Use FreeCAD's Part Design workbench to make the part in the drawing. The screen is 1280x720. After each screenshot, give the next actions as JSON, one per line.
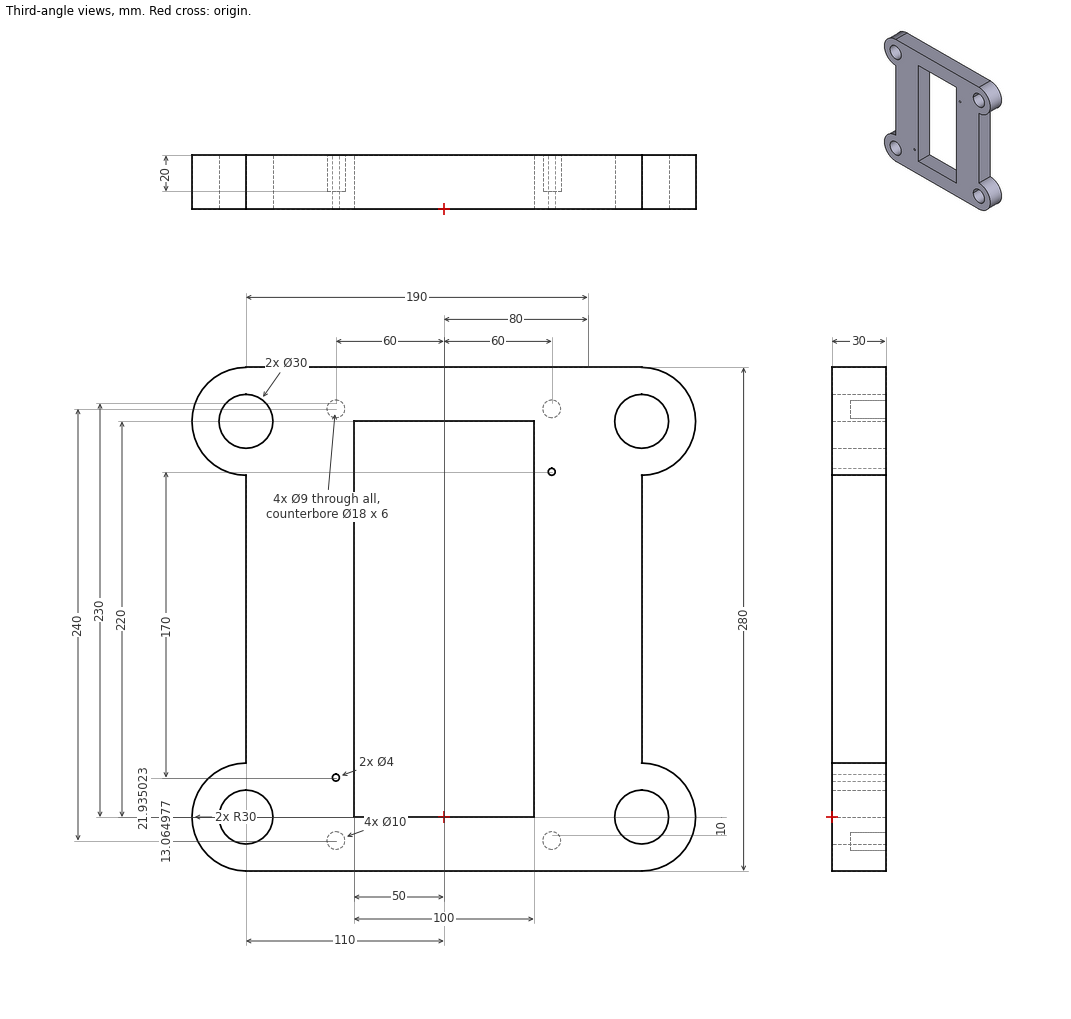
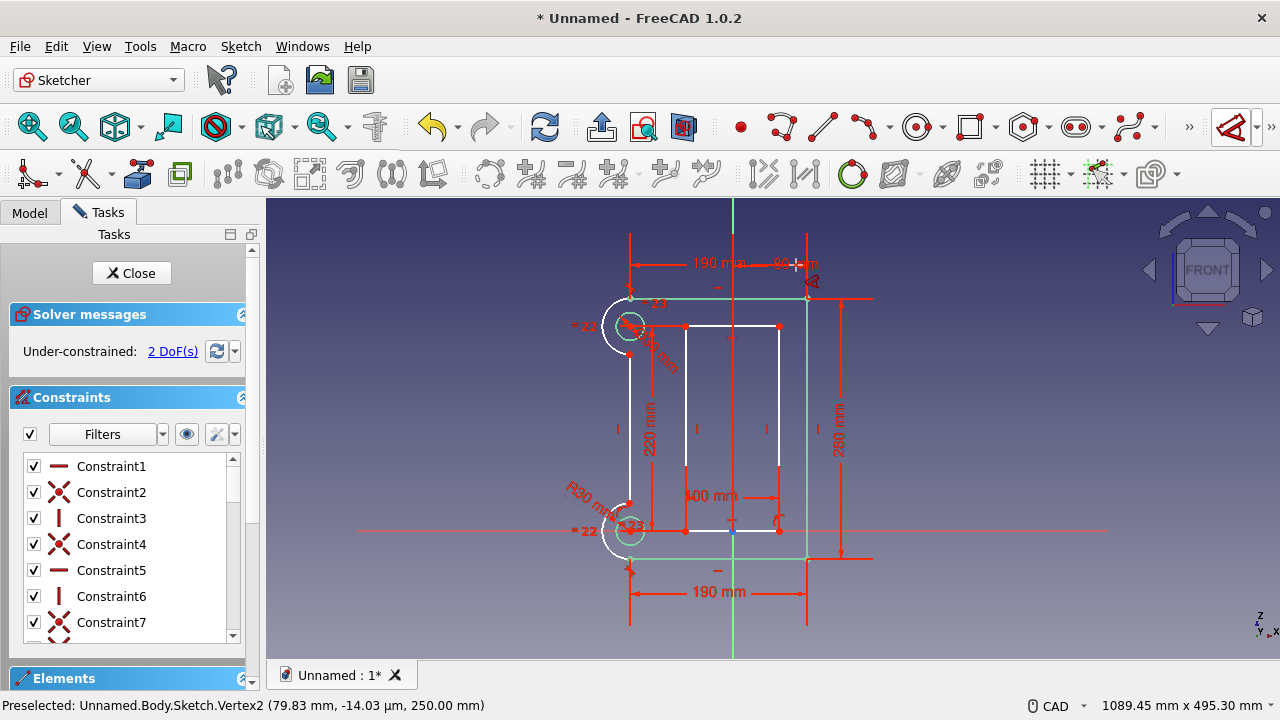
{"action": "left_click", "coordinate": [686, 326]}
{"action": "left_click", "coordinate": [709, 613]}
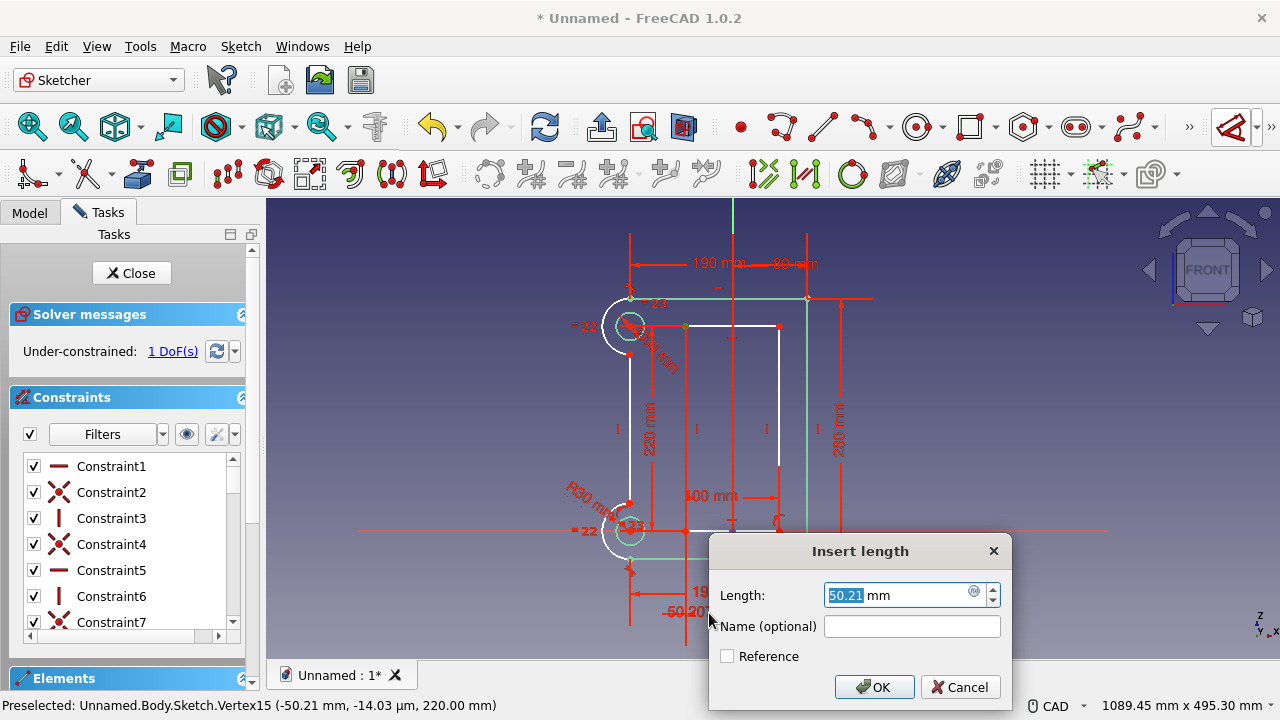
{"action": "type", "text": "50"}
{"action": "key", "text": "Return"}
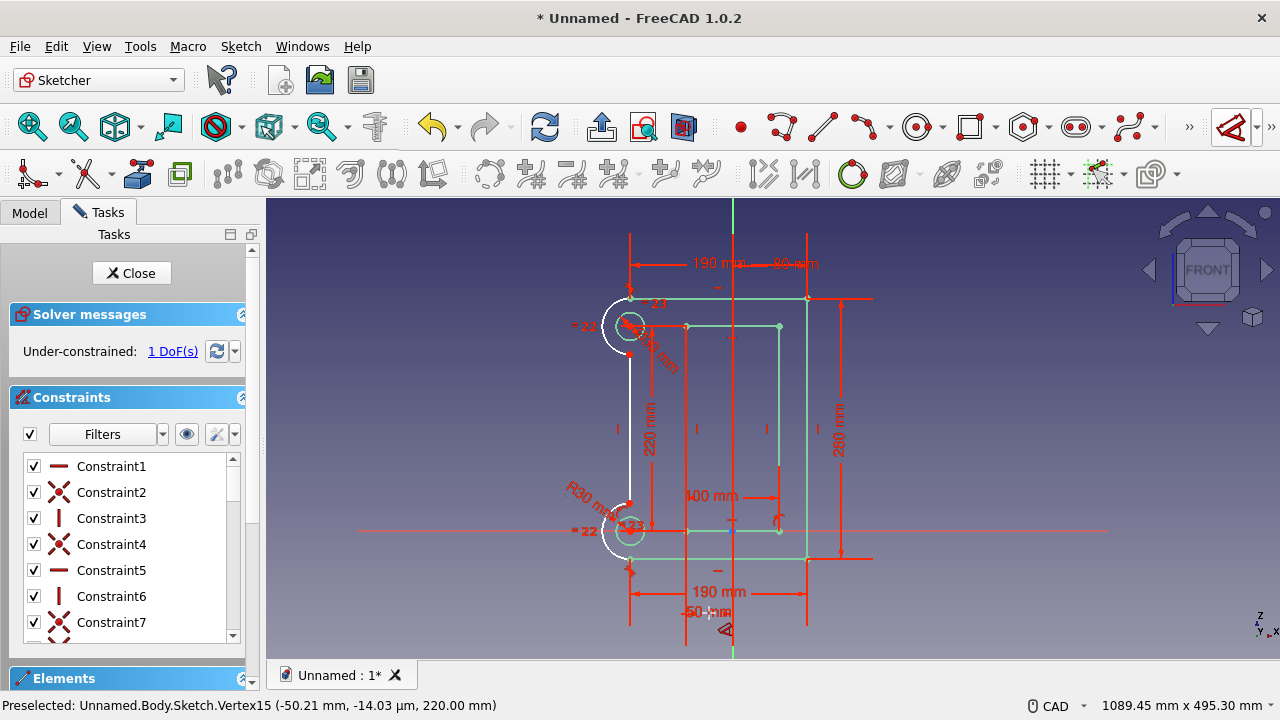
{"action": "left_click", "coordinate": [630, 503]}
{"action": "left_click", "coordinate": [658, 469]}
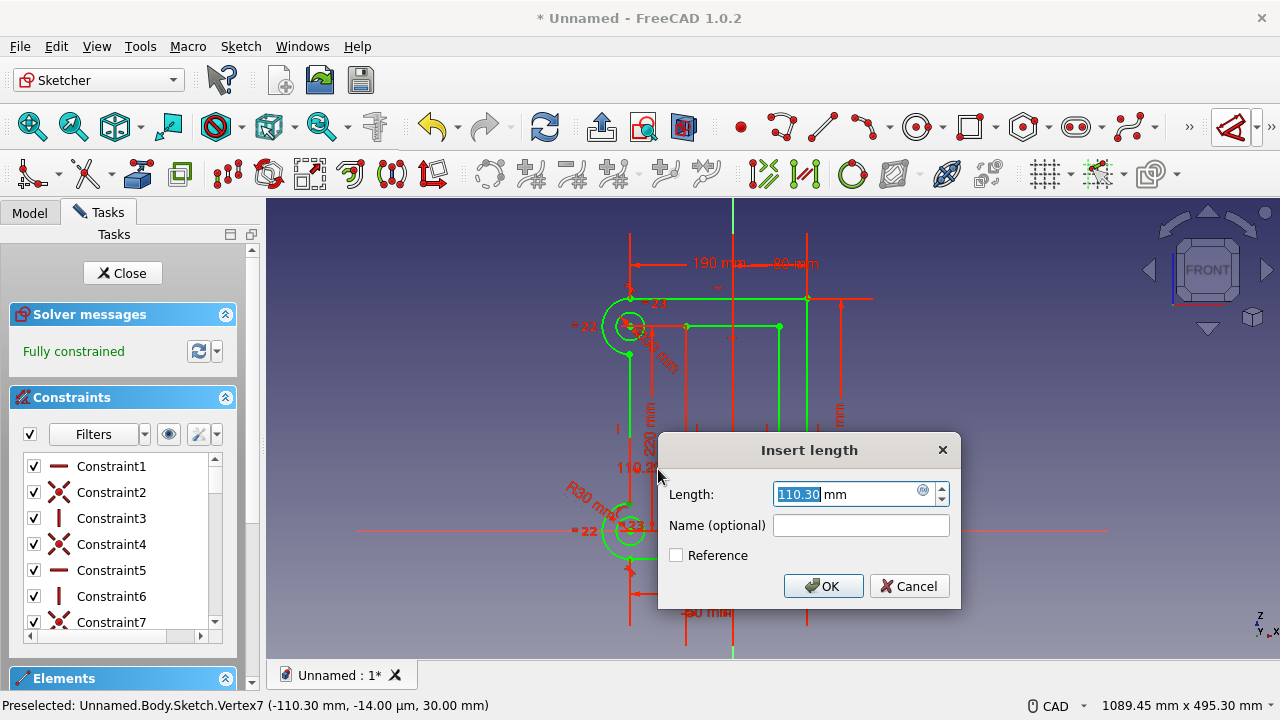
{"action": "type", "text": "110"}
{"action": "key", "text": "Return"}
{"action": "key", "text": "Escape"}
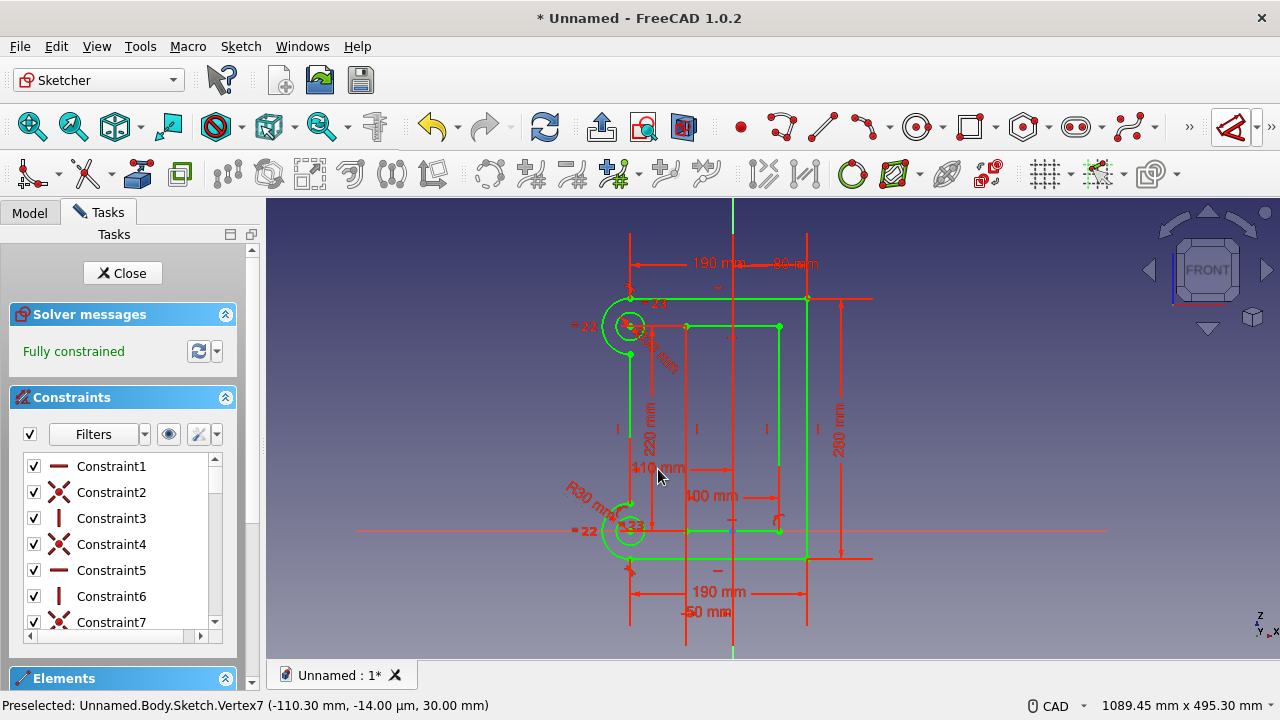
{"action": "left_click", "coordinate": [123, 273]}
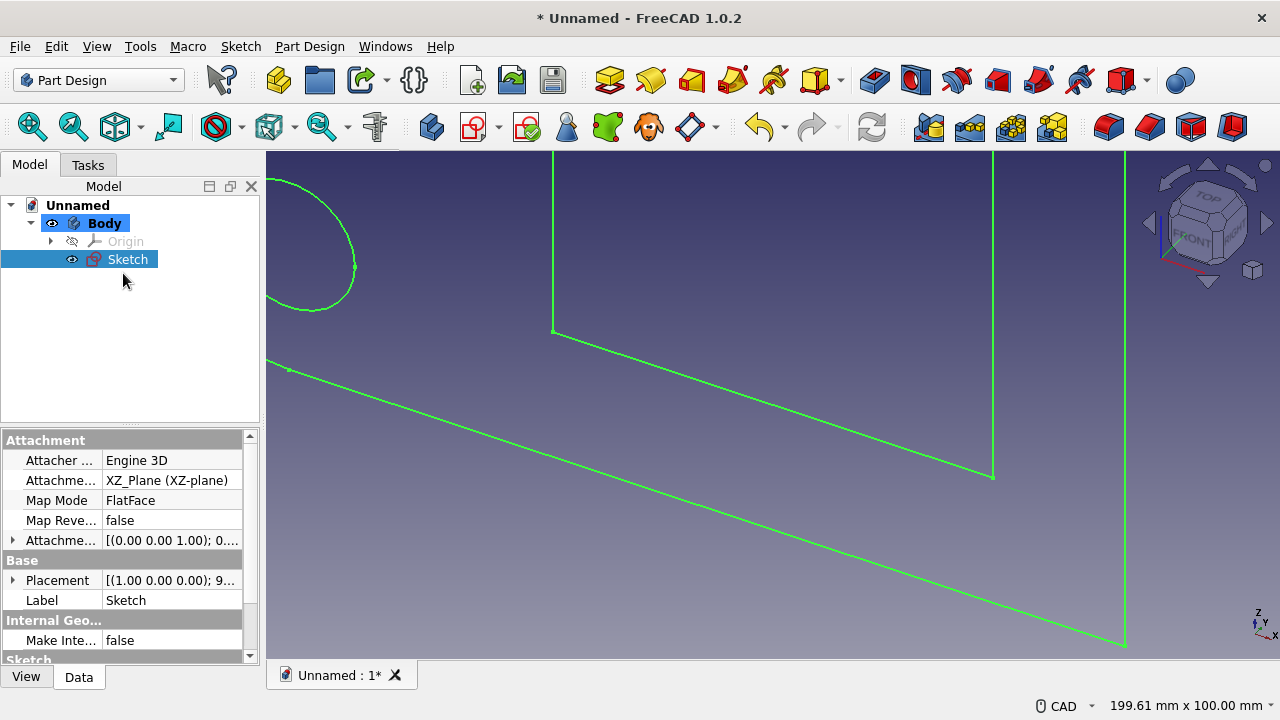
{"action": "left_click", "coordinate": [610, 80]}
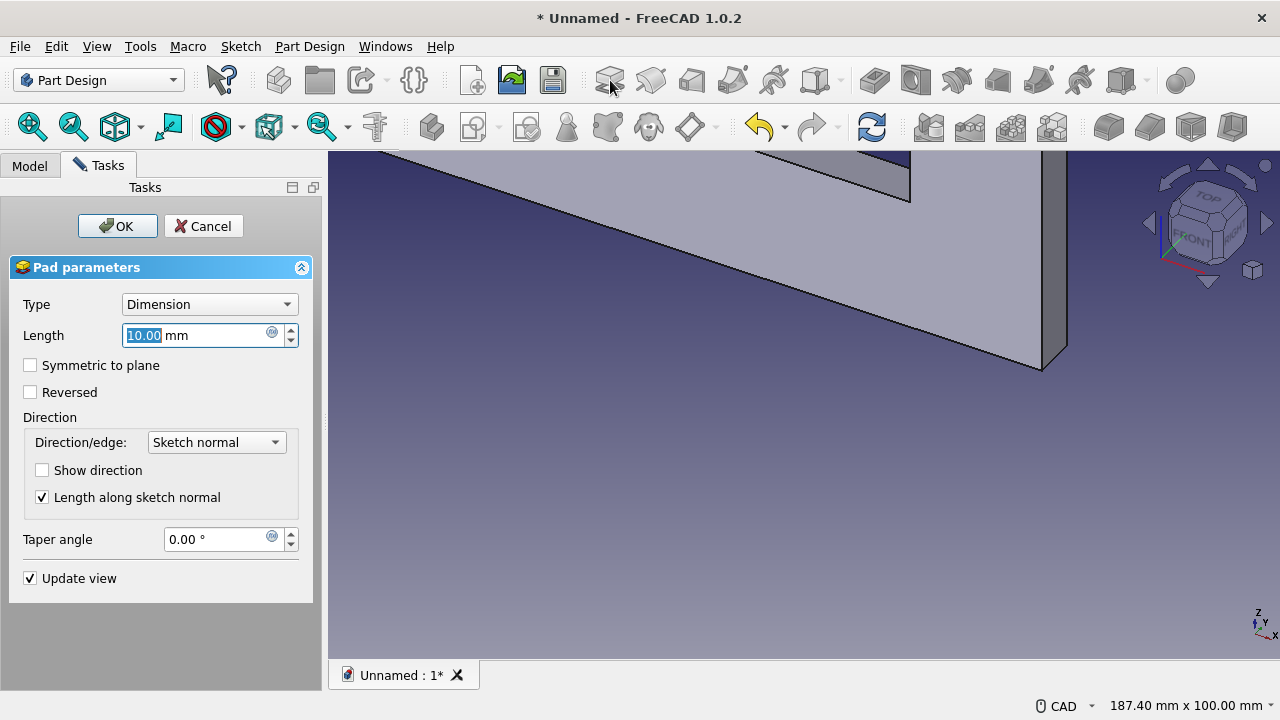
{"action": "type", "text": "30"}
{"action": "key", "text": "Tab"}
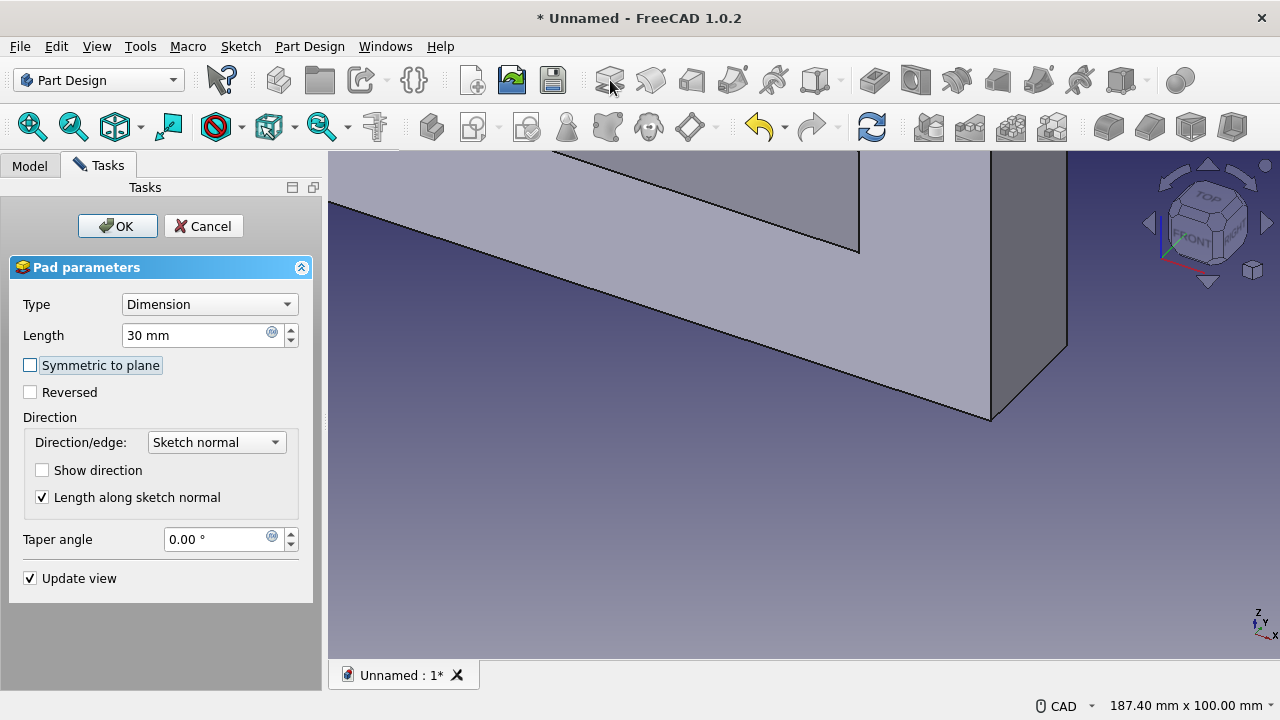
{"action": "left_click", "coordinate": [31, 392]}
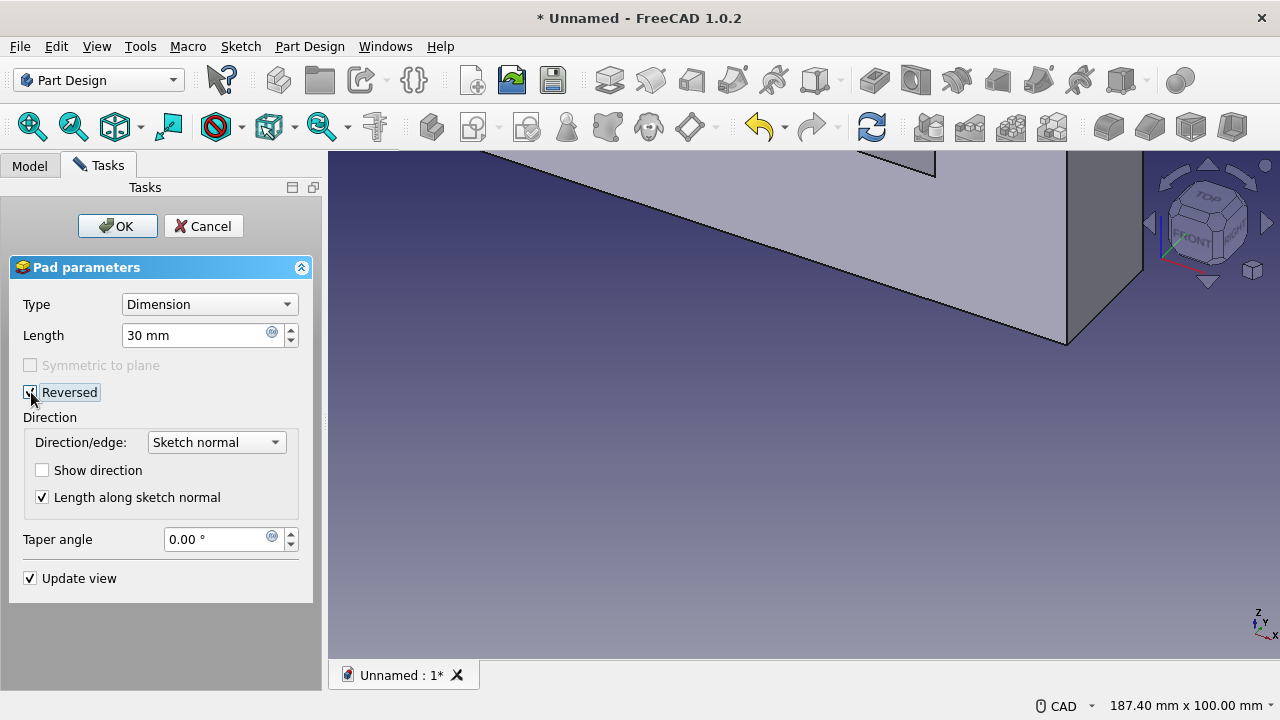
{"action": "left_click", "coordinate": [118, 226]}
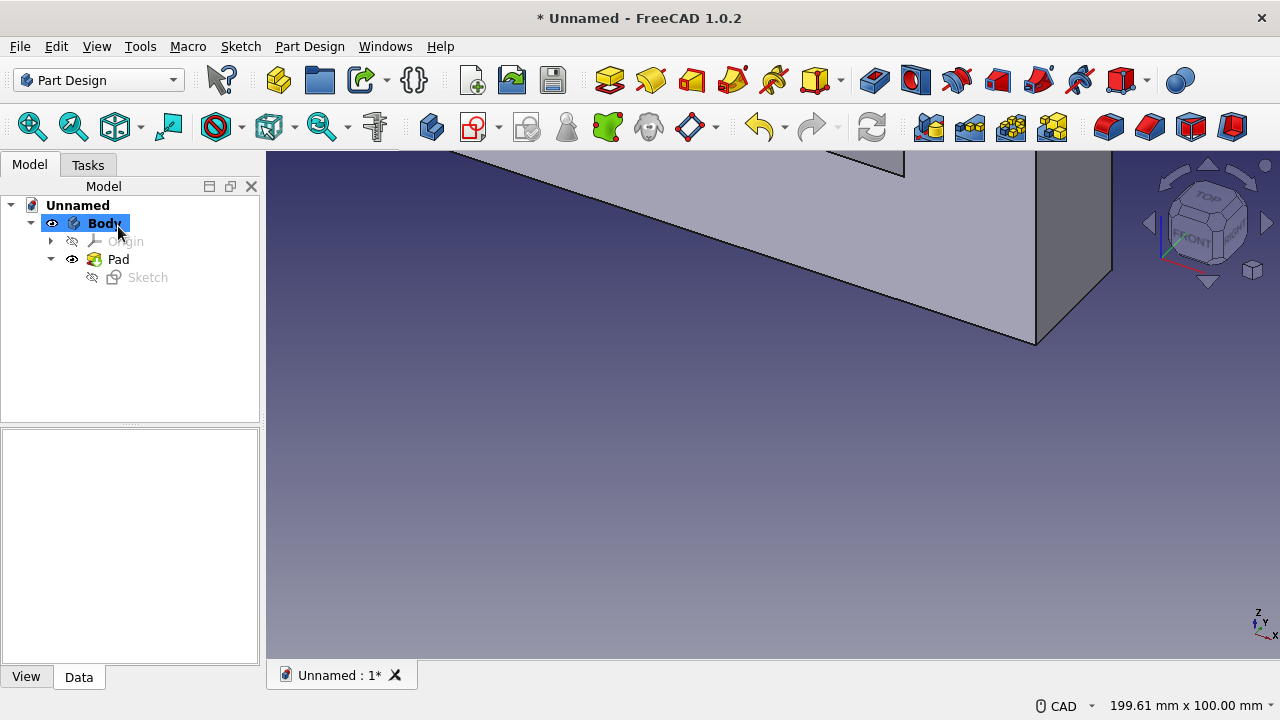
{"action": "key", "text": "v f"}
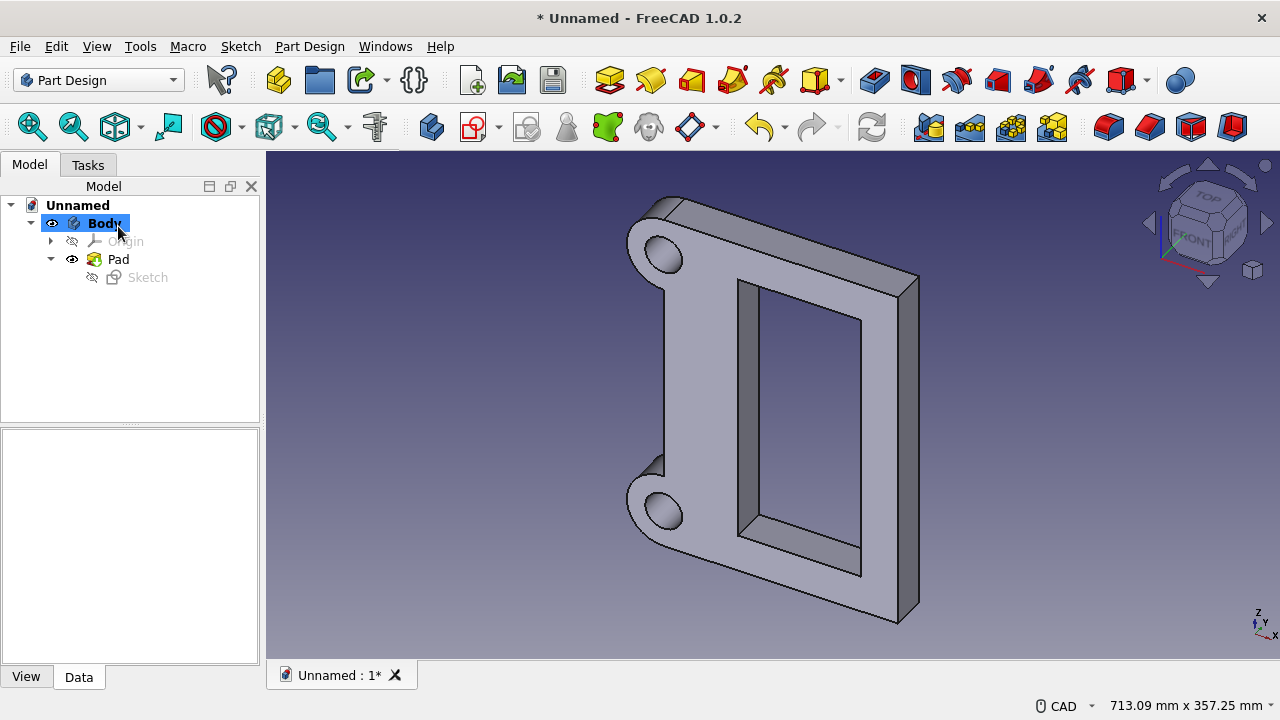
{"action": "left_click", "coordinate": [685, 296]}